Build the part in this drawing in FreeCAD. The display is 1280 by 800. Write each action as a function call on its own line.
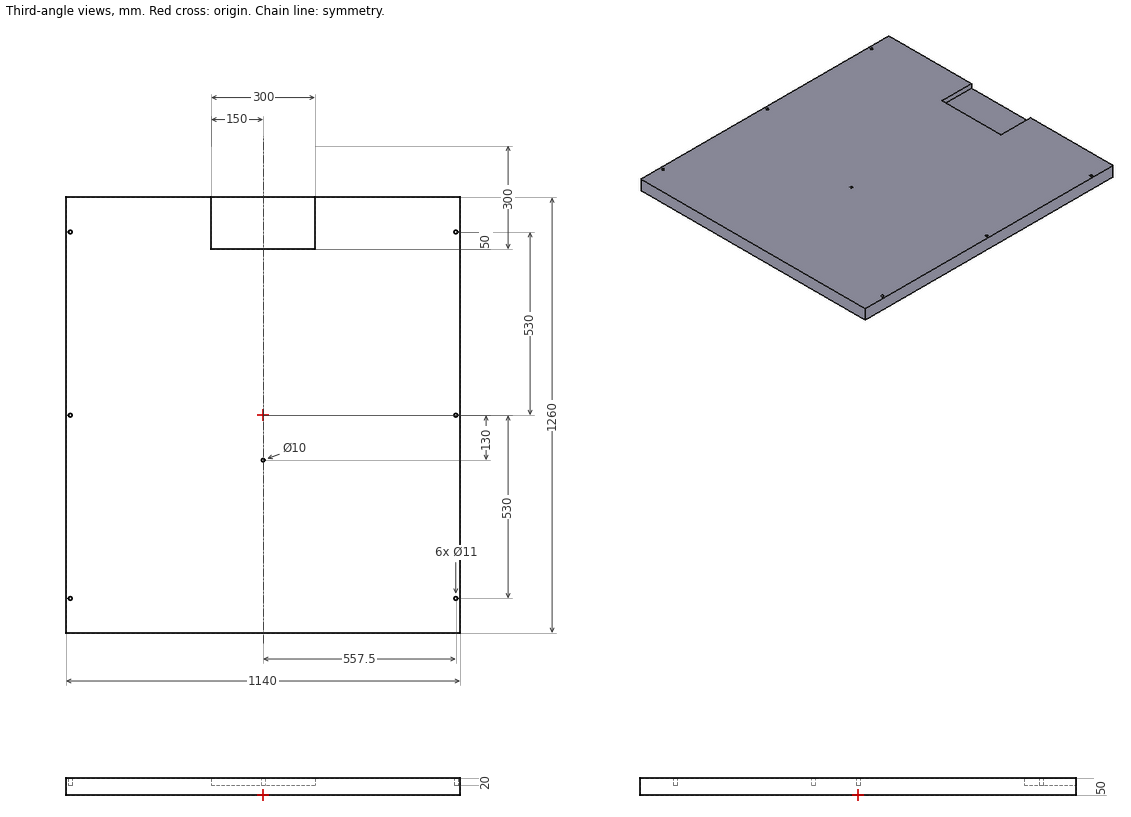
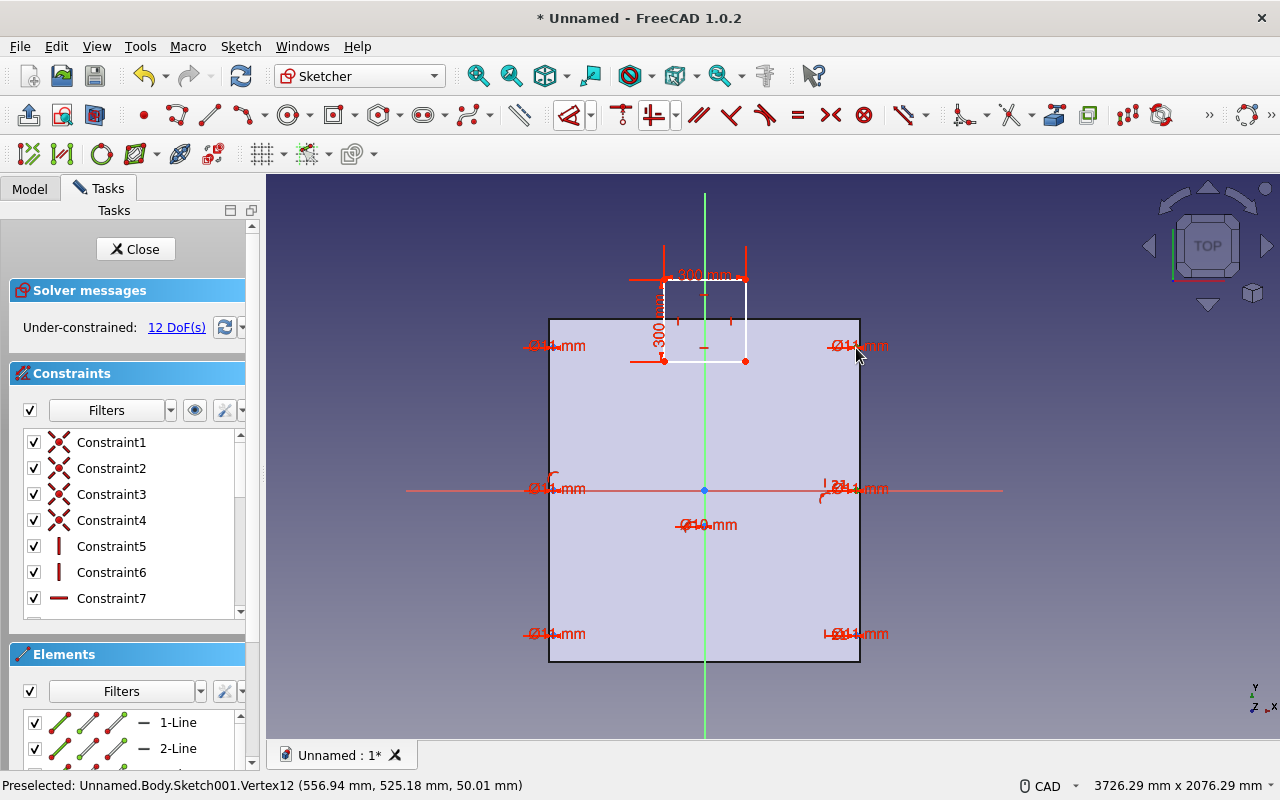
key(v)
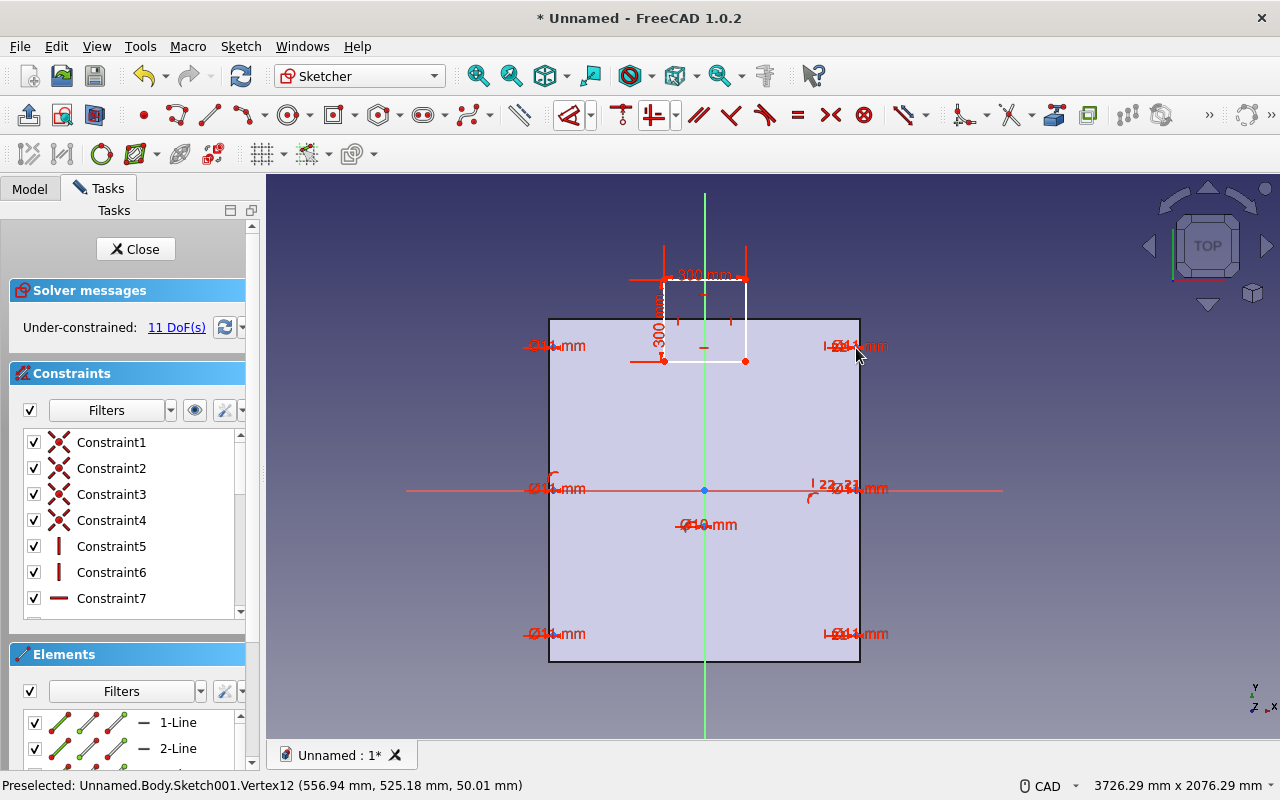
click(553, 348)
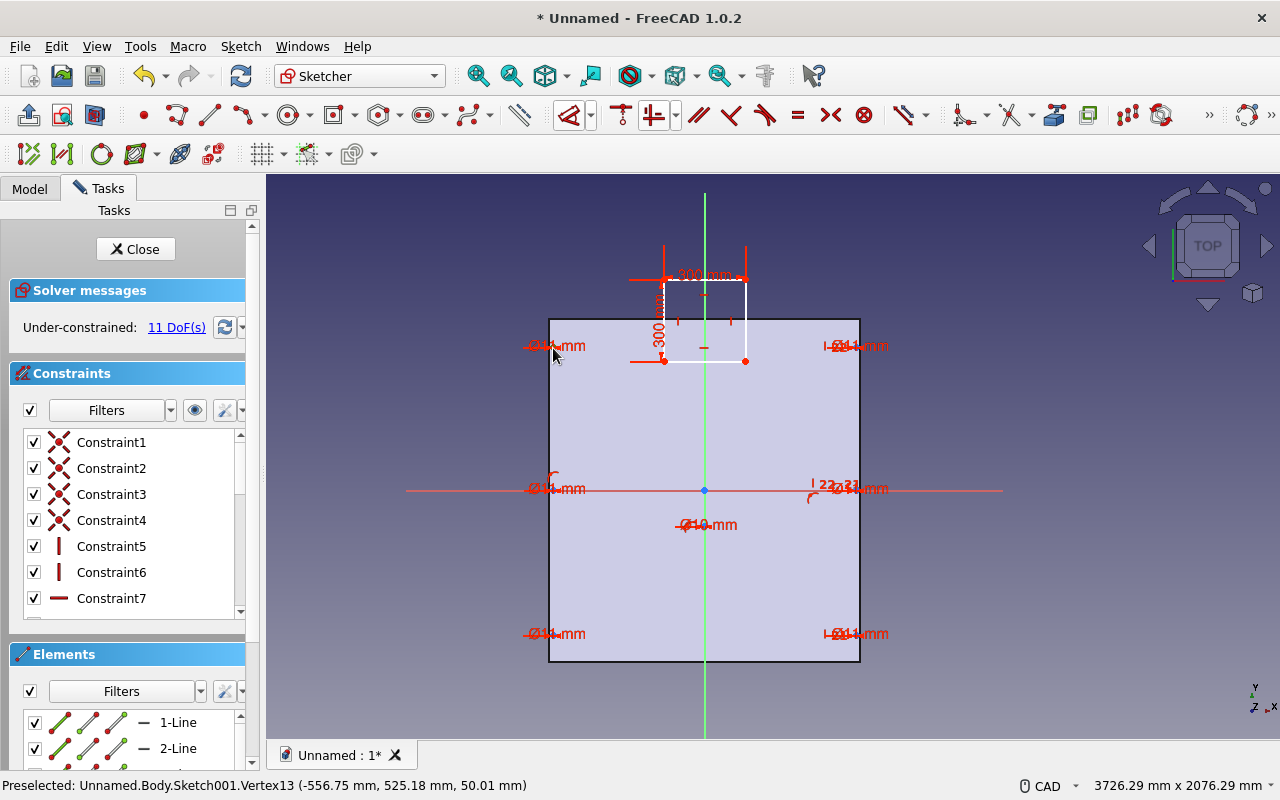
click(553, 491)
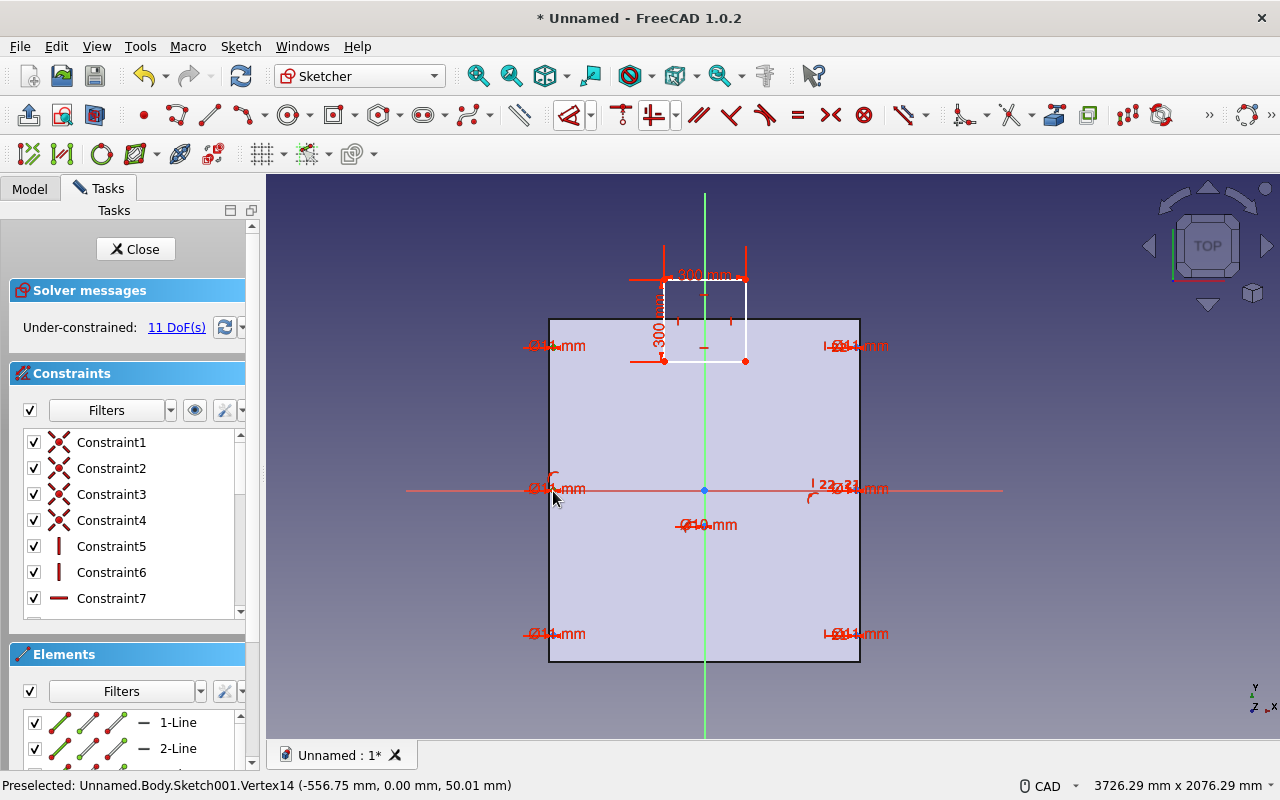
click(676, 116)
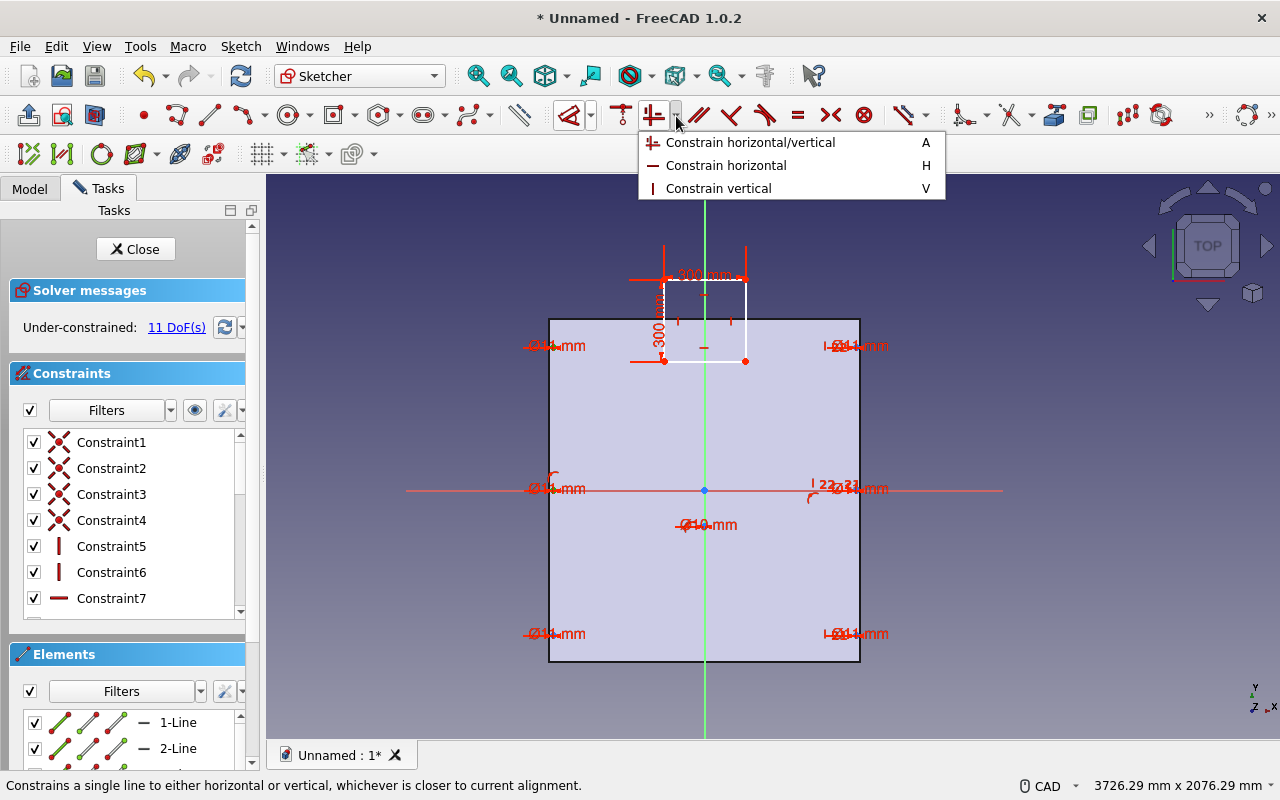
click(792, 188)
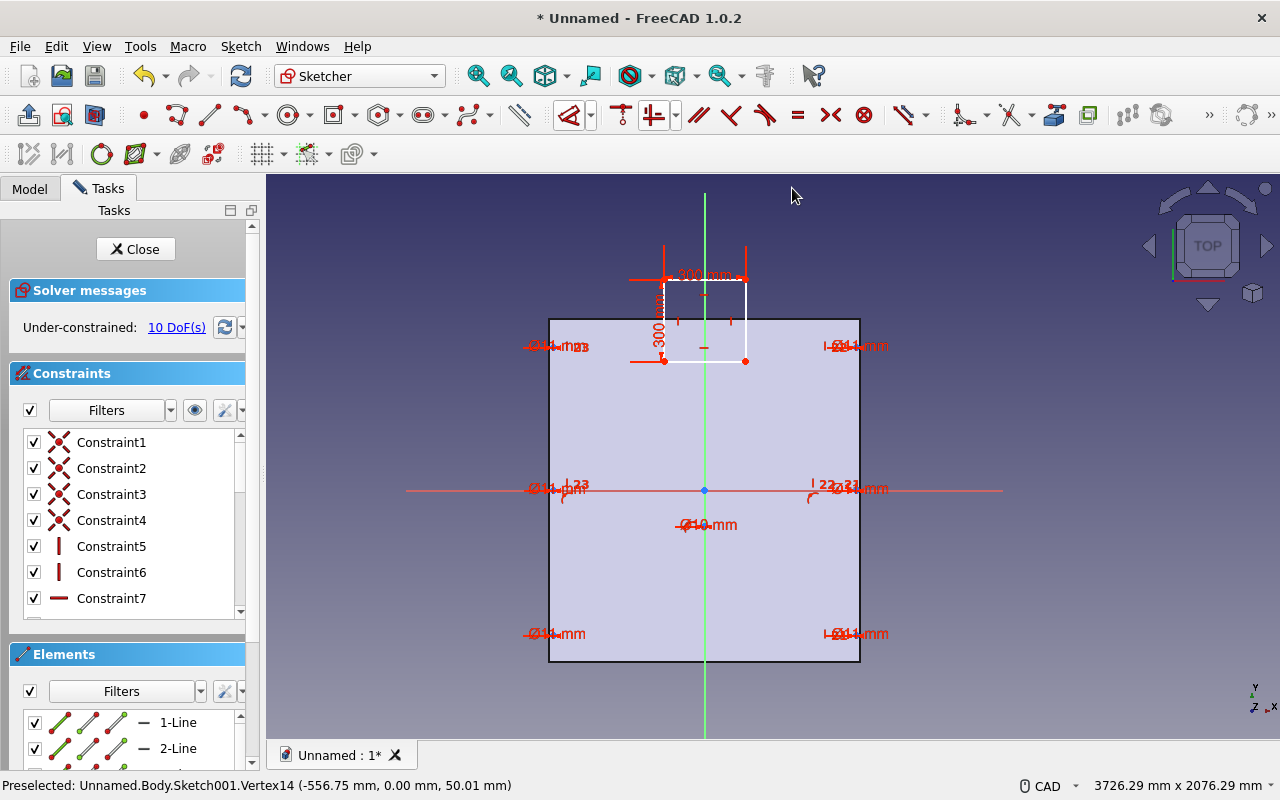
click(553, 491)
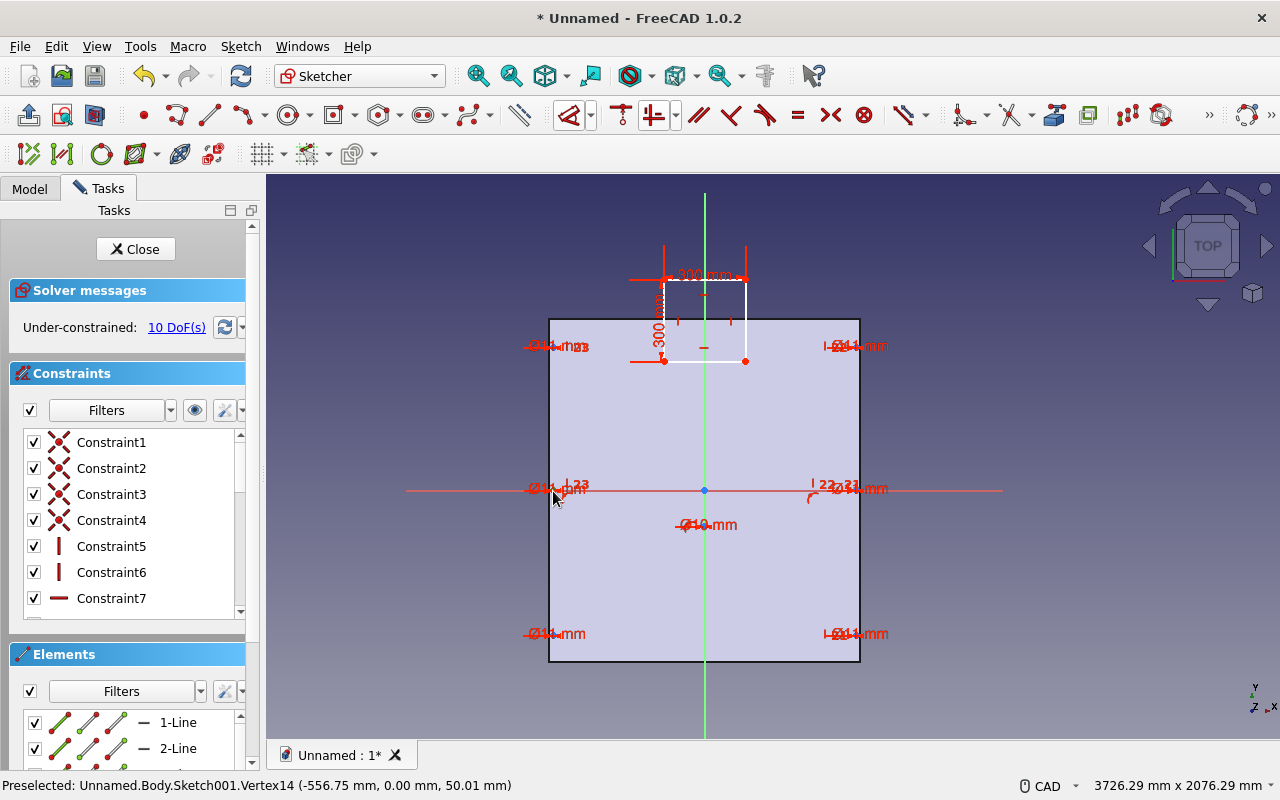
click(553, 636)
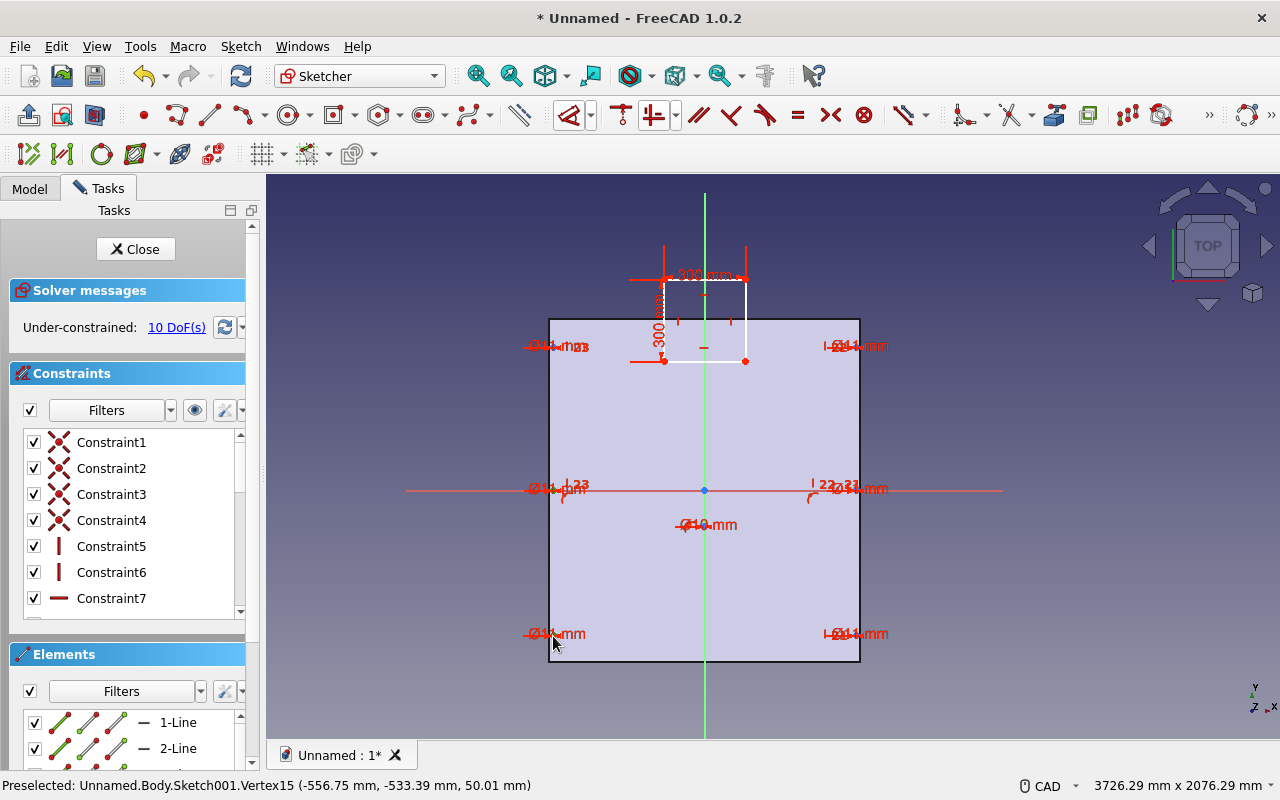
click(676, 116)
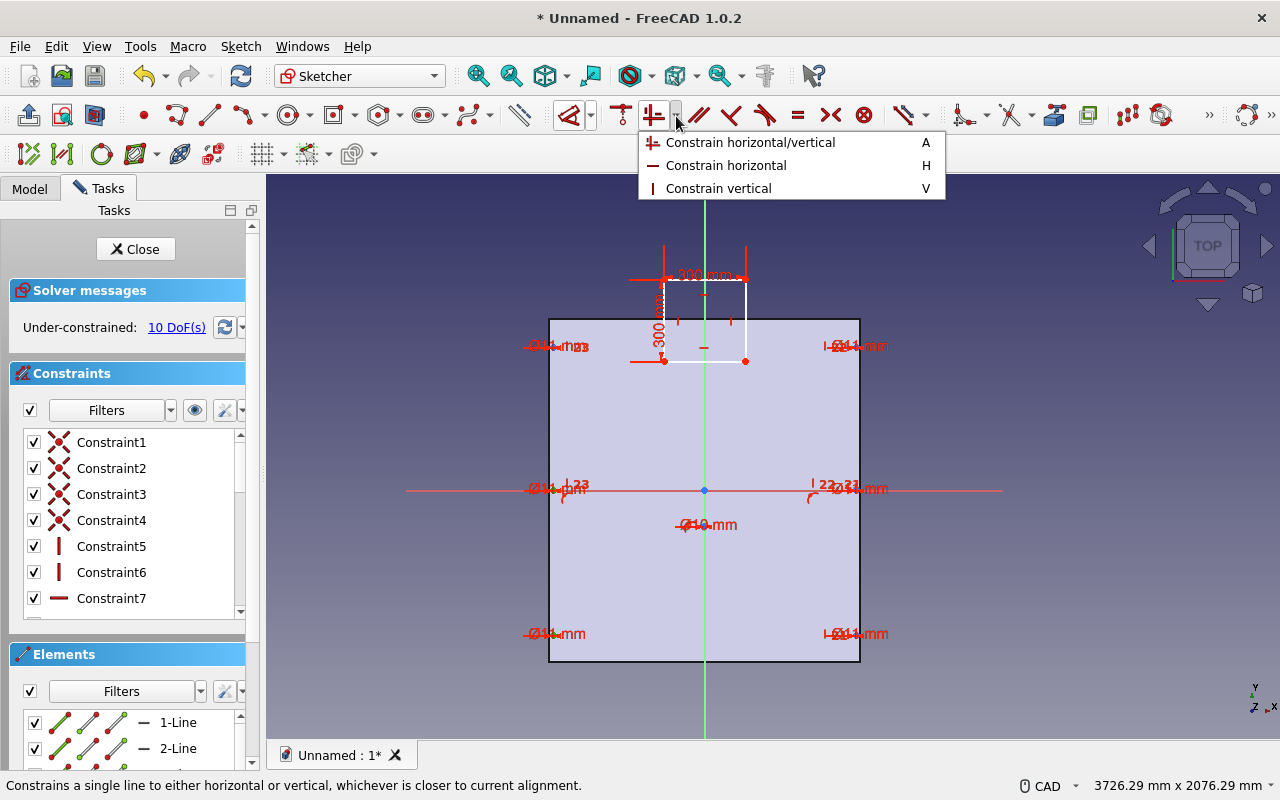
click(792, 188)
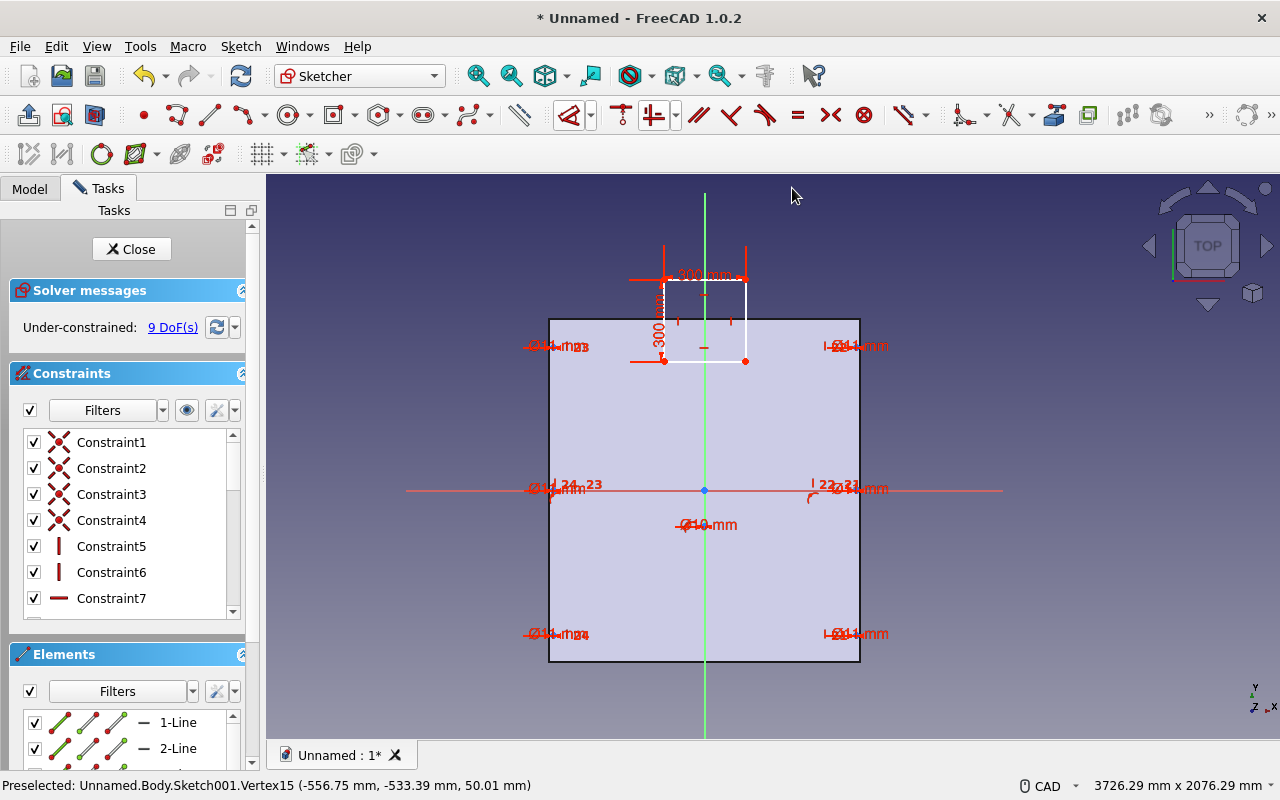
click(856, 636)